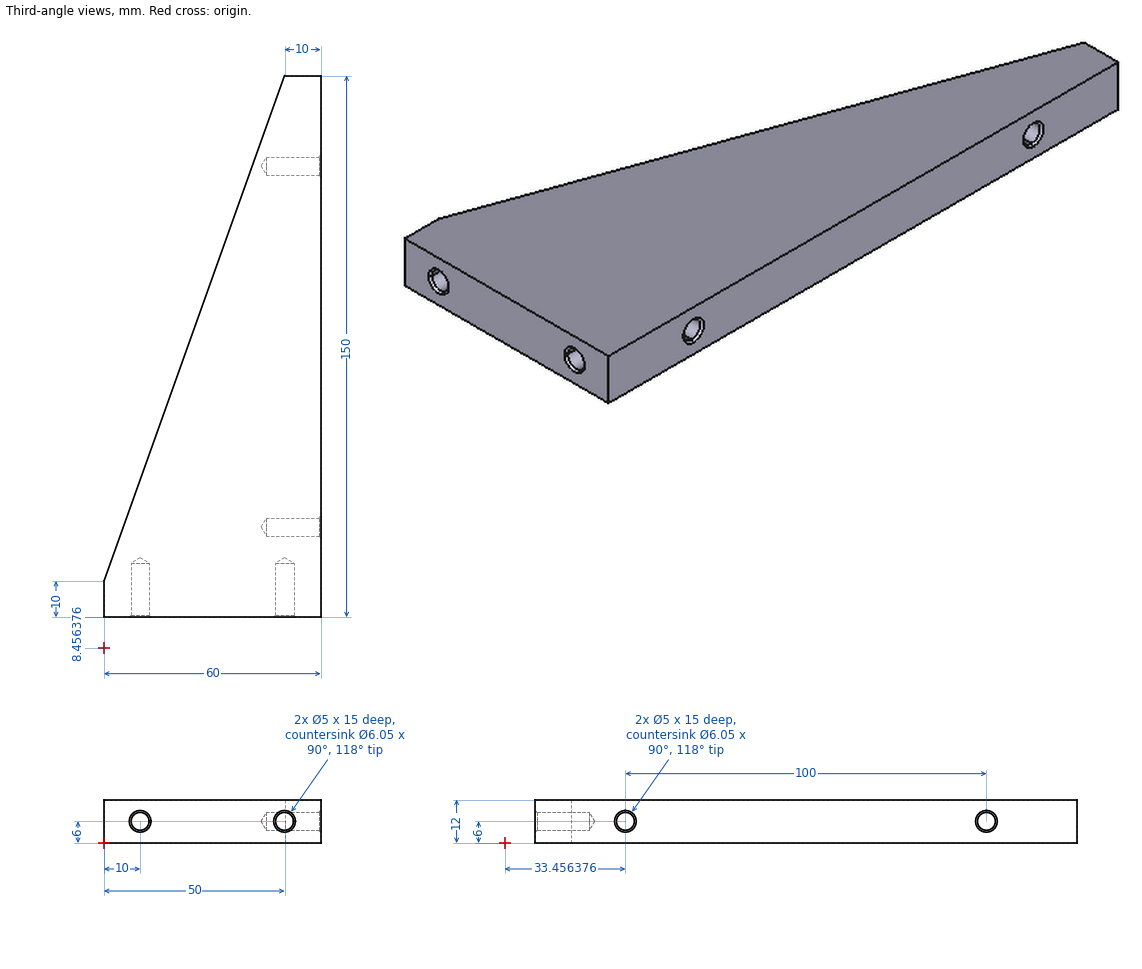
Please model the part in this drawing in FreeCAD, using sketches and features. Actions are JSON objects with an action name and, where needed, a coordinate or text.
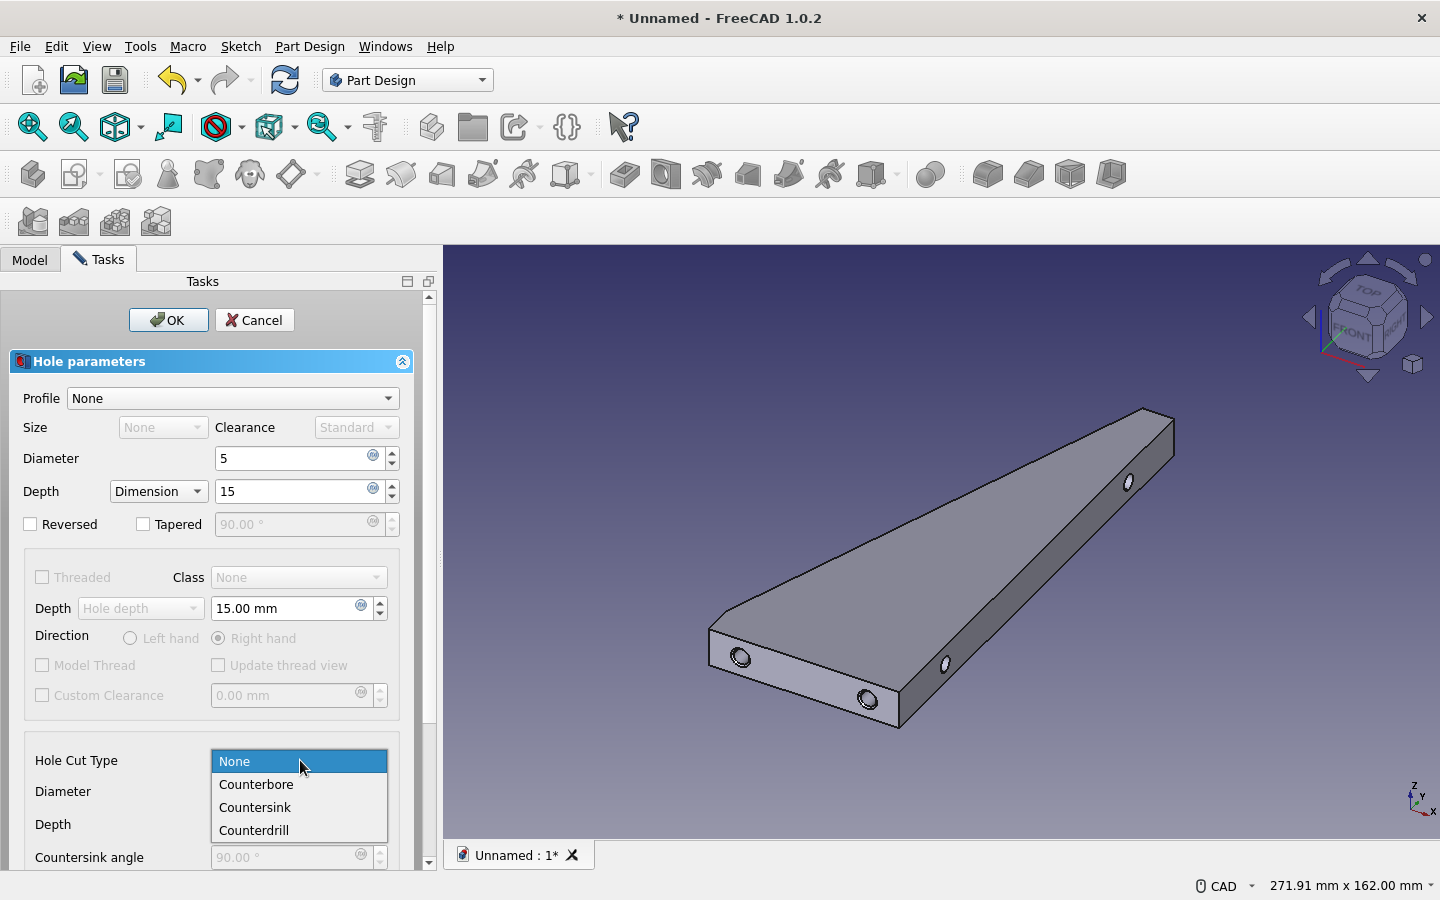
{"action": "left_click", "coordinate": [298, 808]}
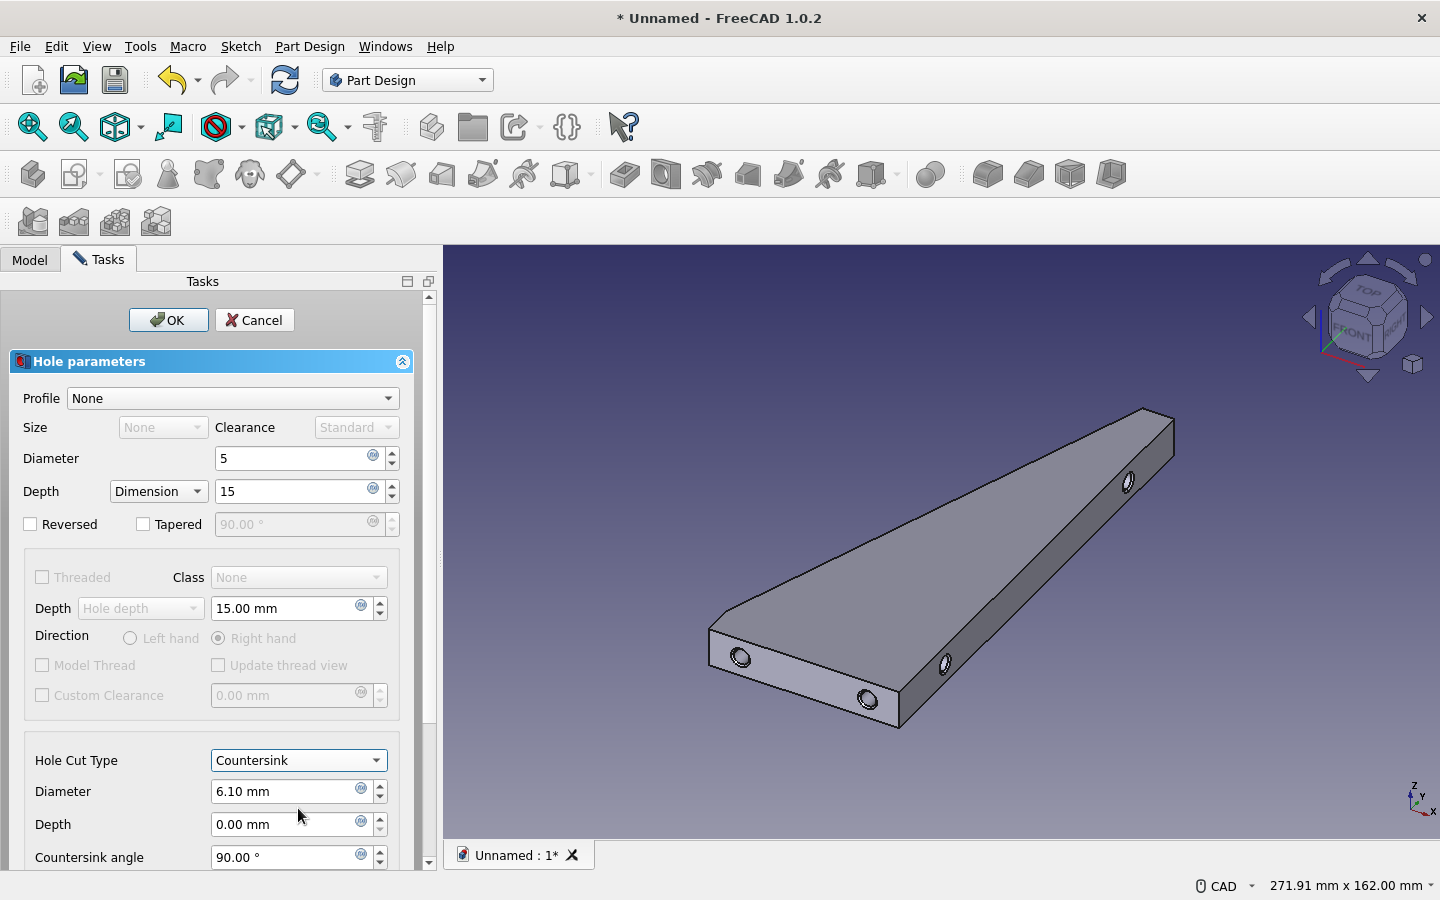
{"action": "triple_click", "coordinate": [292, 792]}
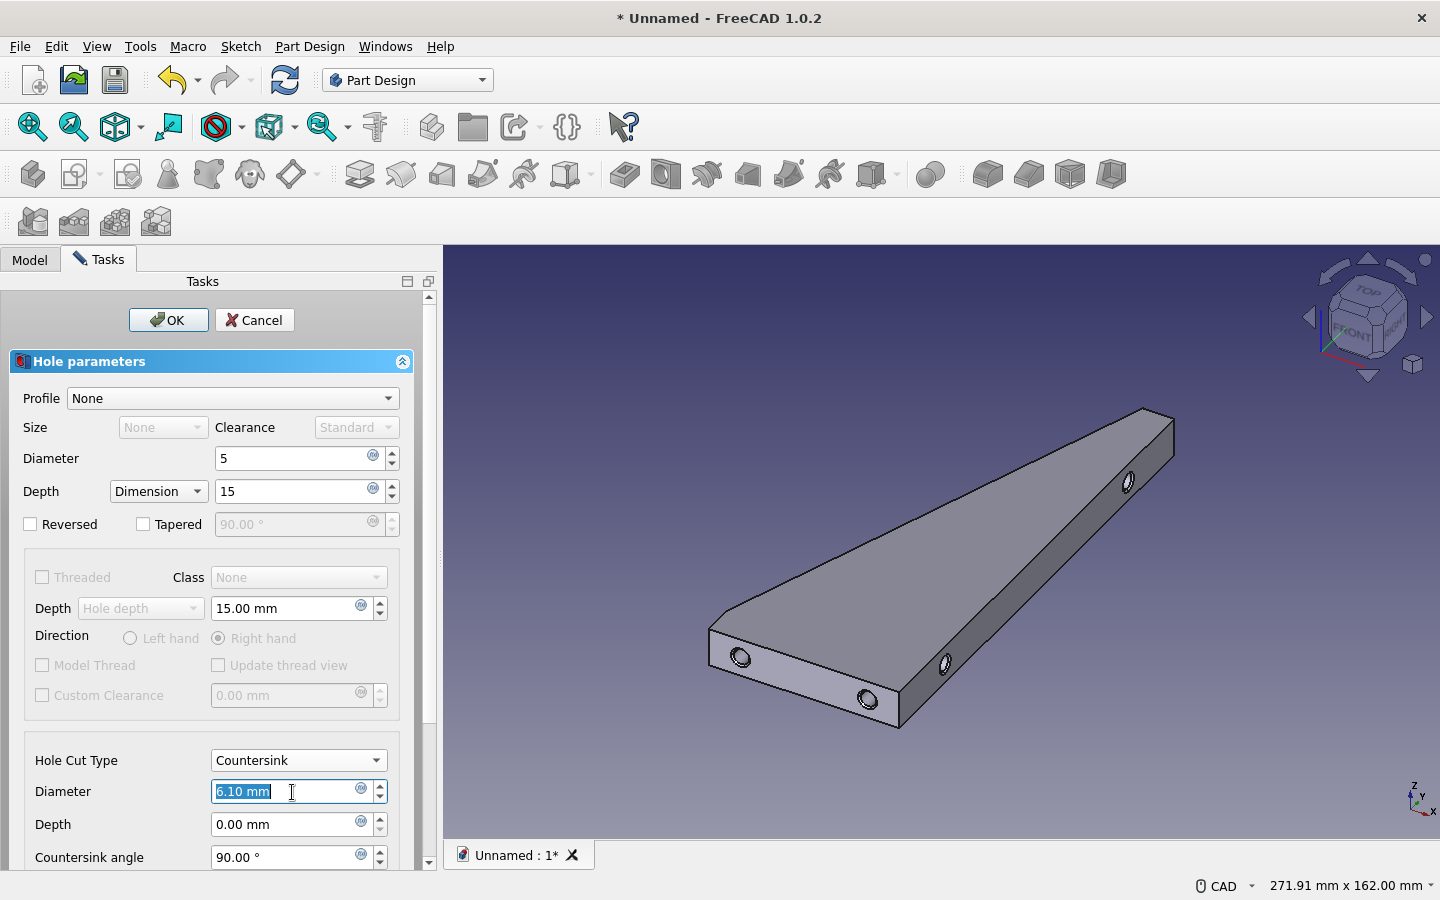
{"action": "type", "text": "6.05"}
{"action": "key", "text": "Tab"}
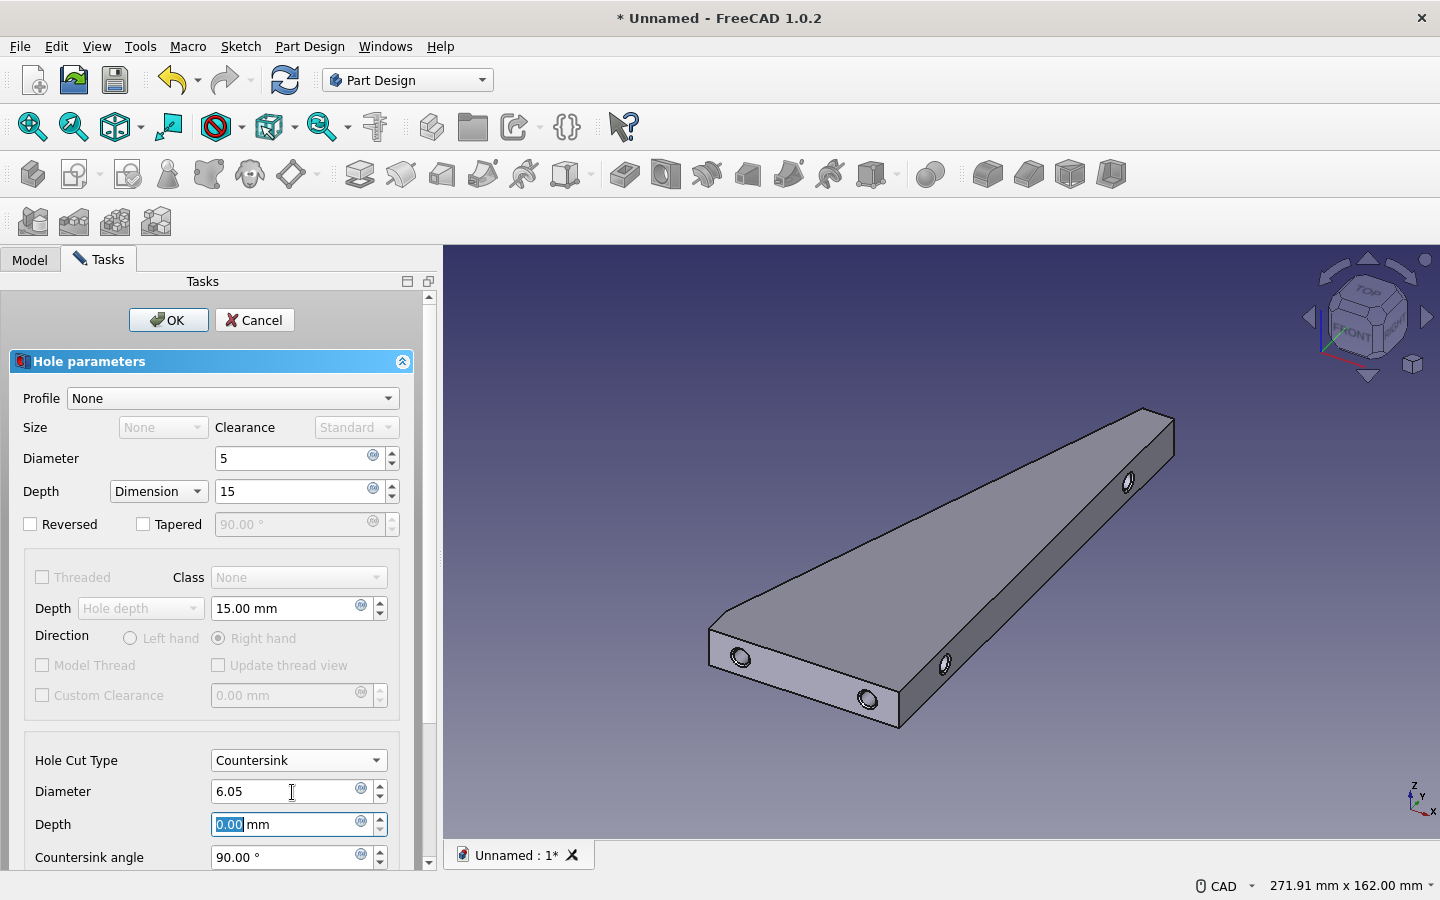
{"action": "left_click", "coordinate": [169, 320]}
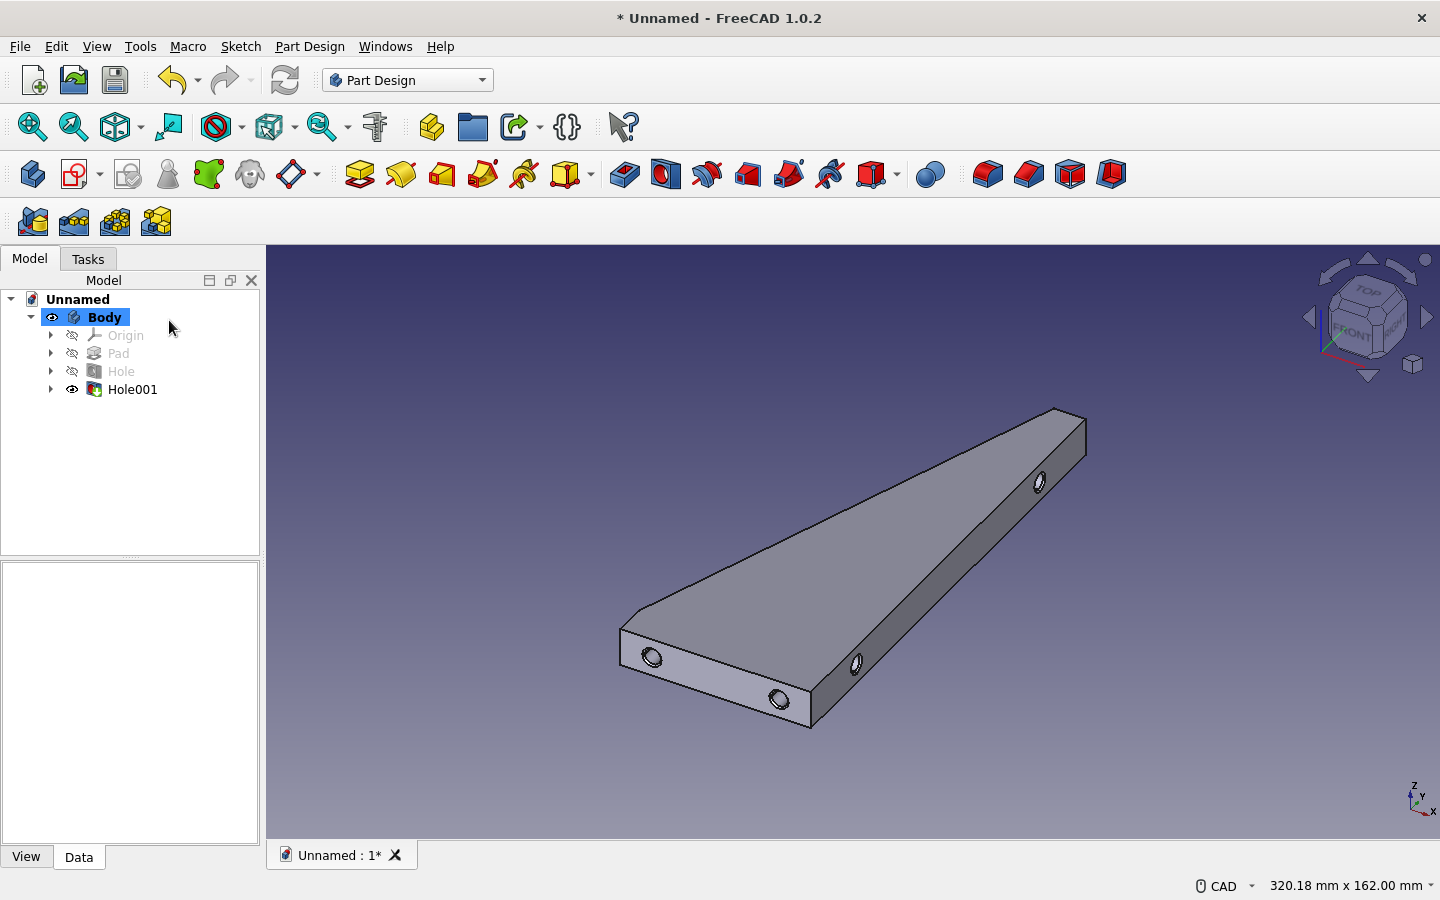
{"action": "key", "text": "0"}